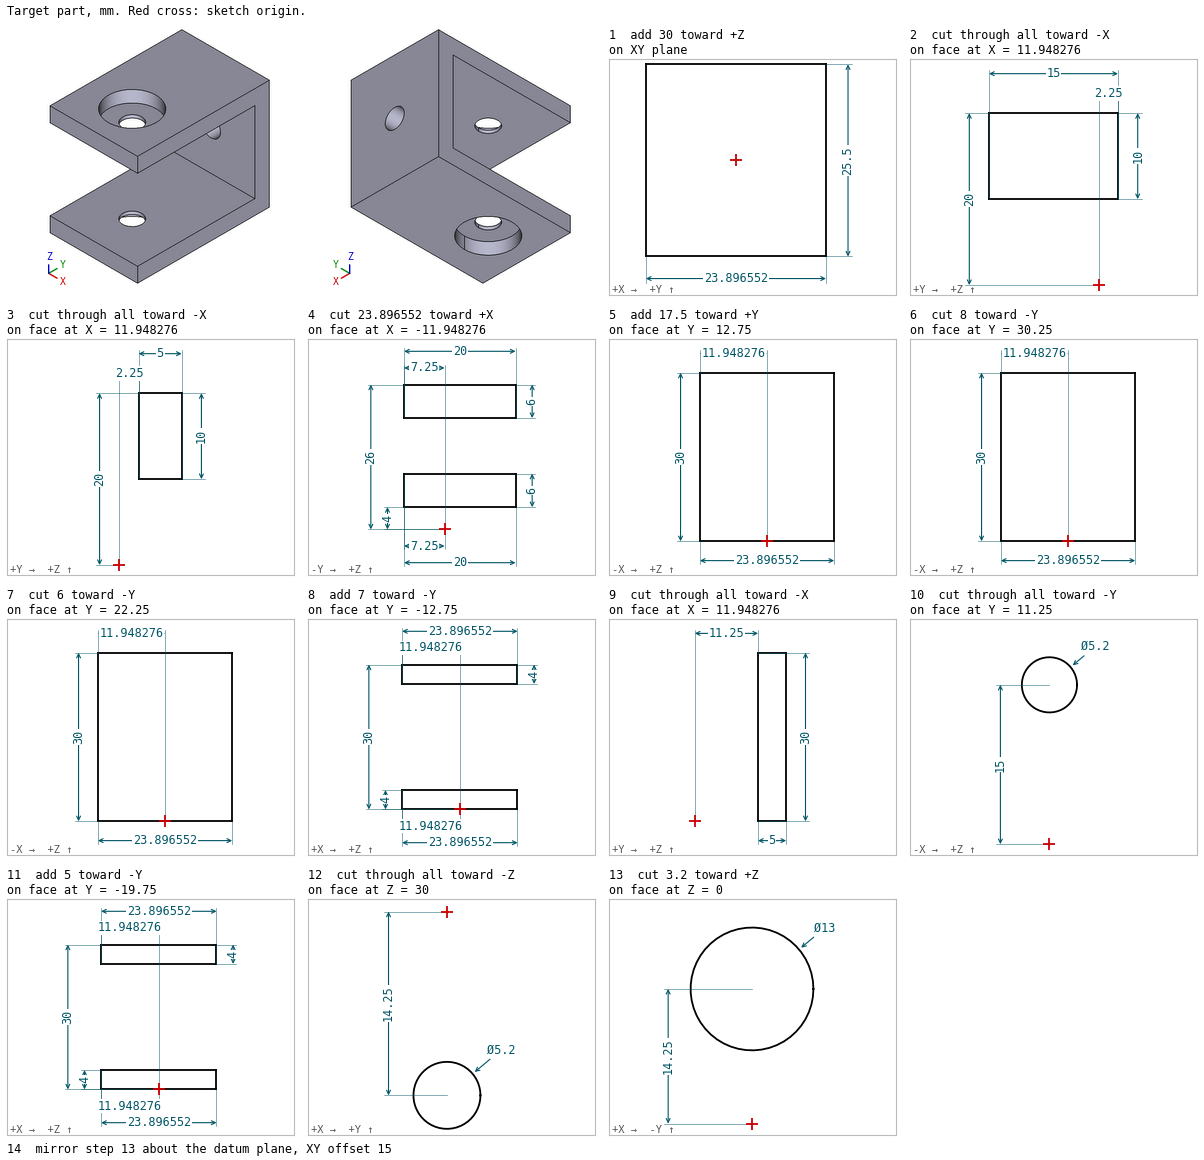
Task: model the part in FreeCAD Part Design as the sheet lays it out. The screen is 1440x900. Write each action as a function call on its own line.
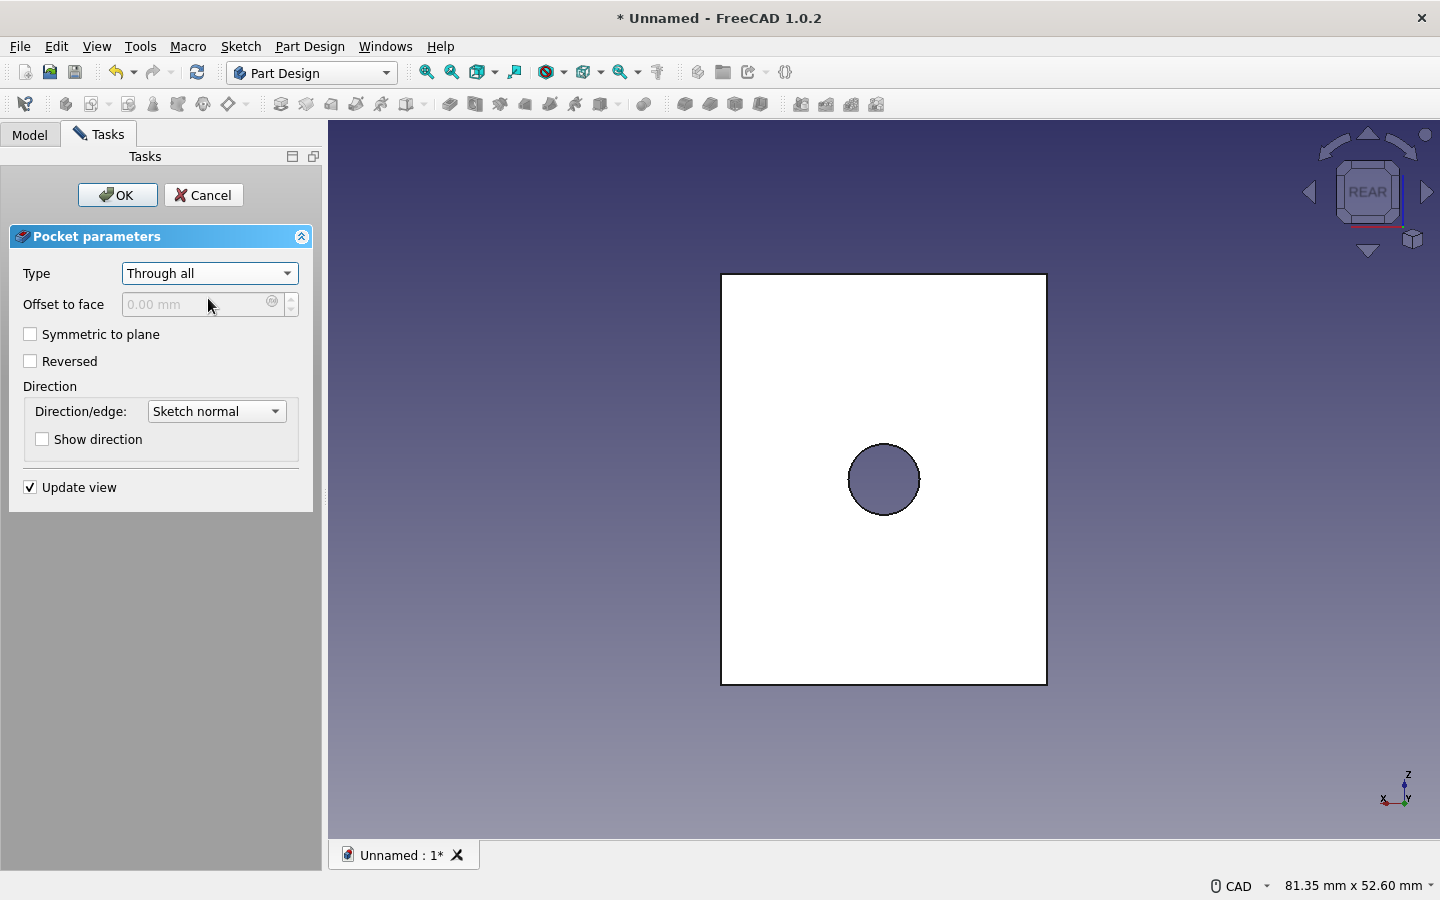
click(118, 195)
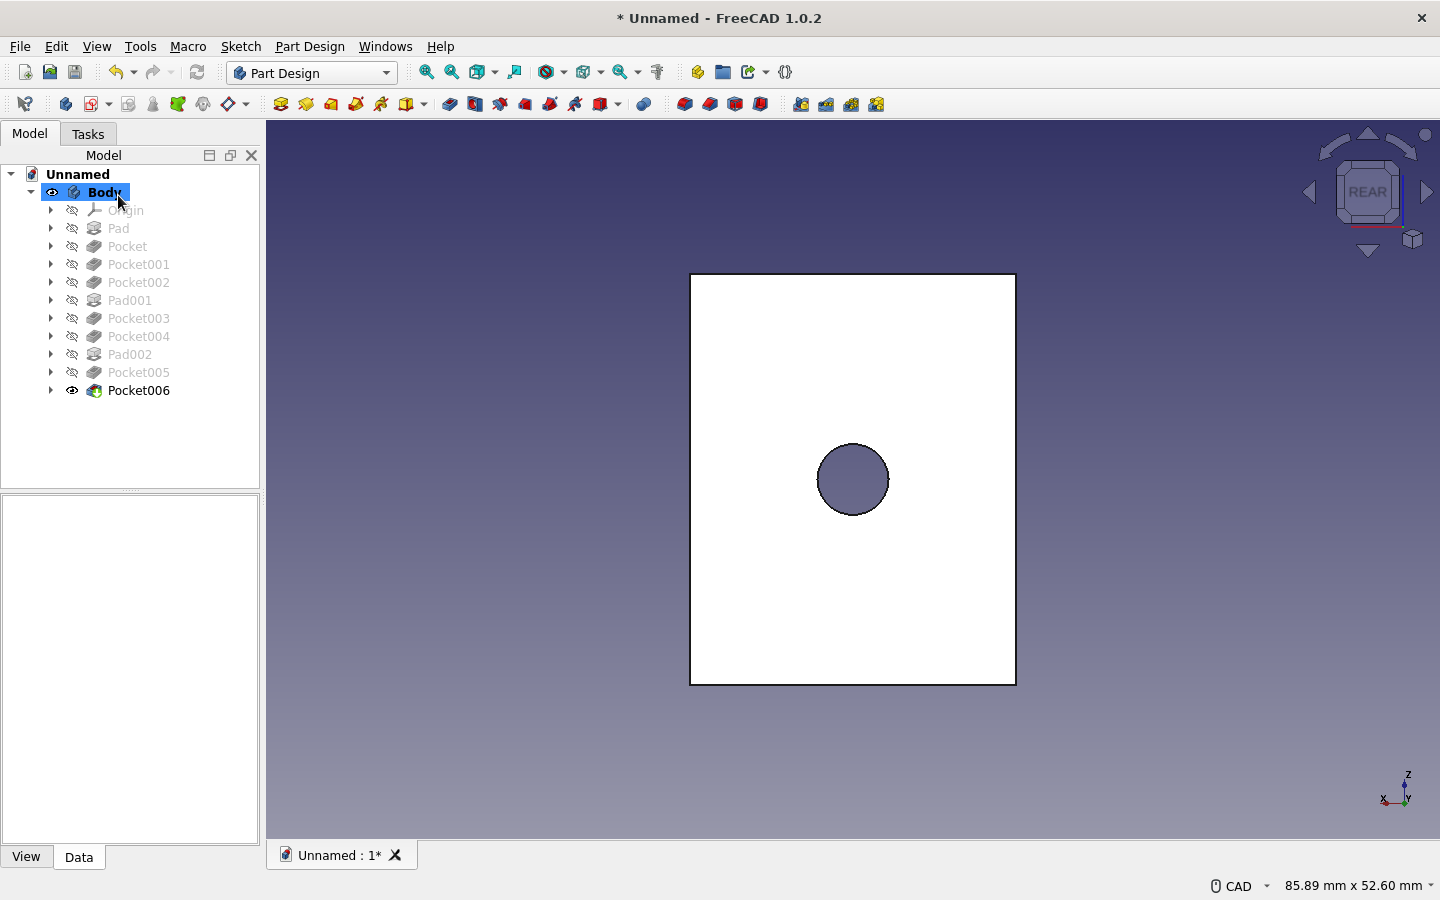
key(0)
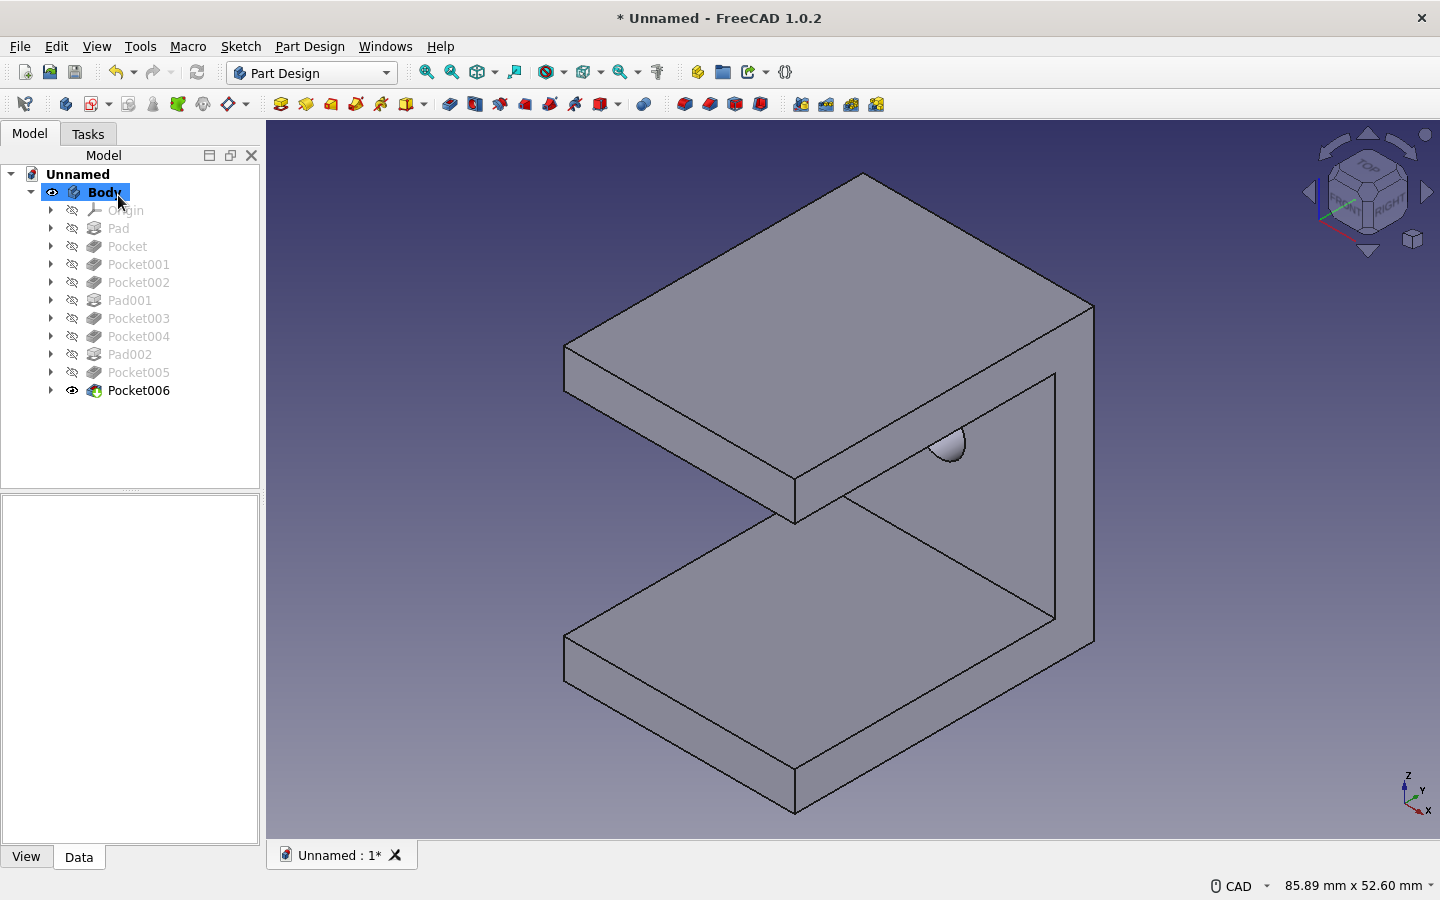
click(745, 472)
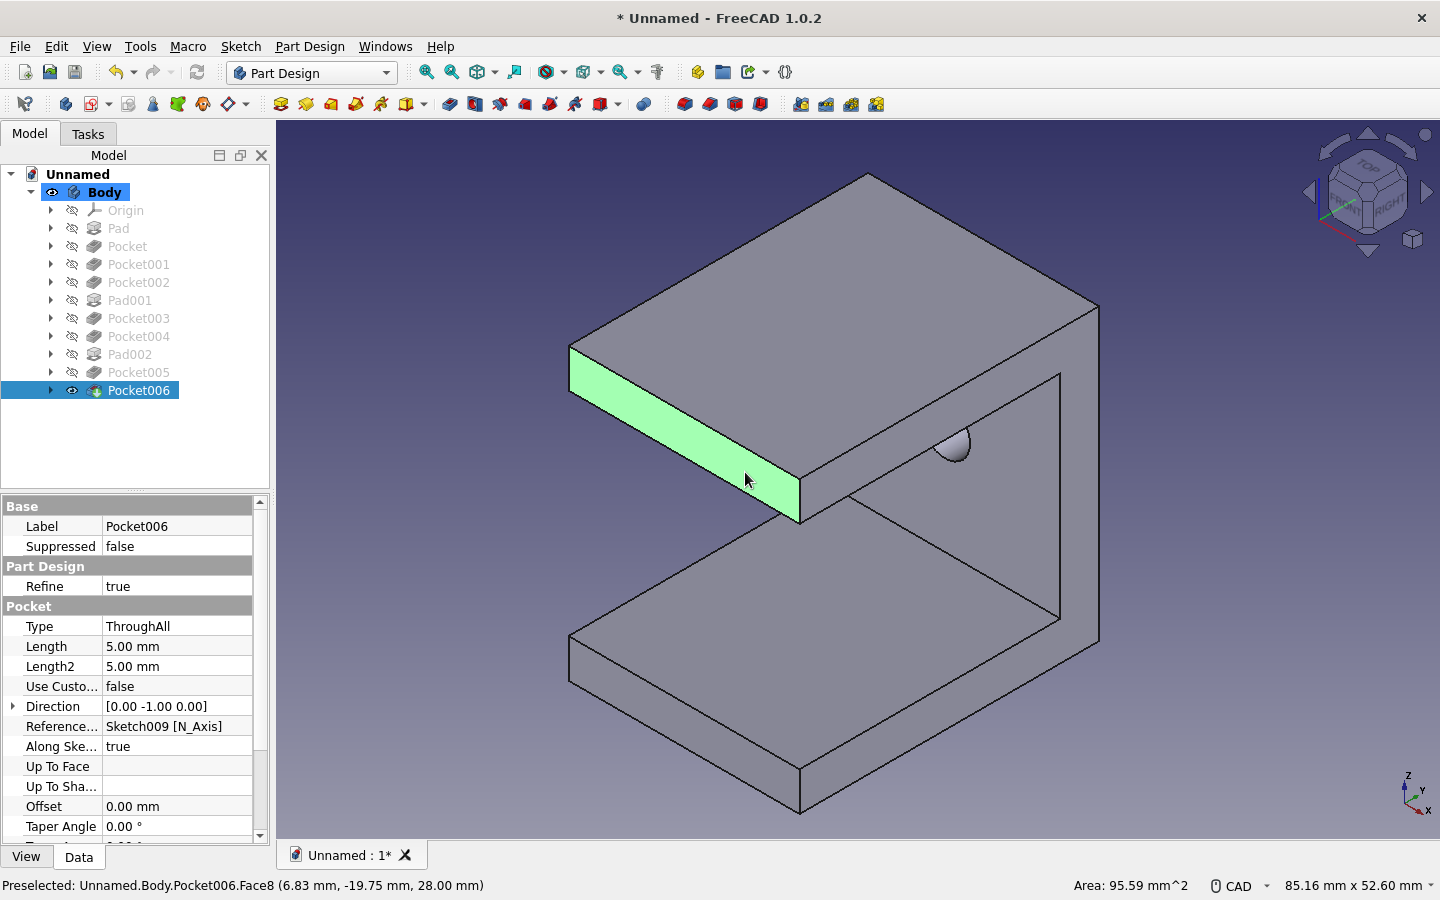
click(90, 104)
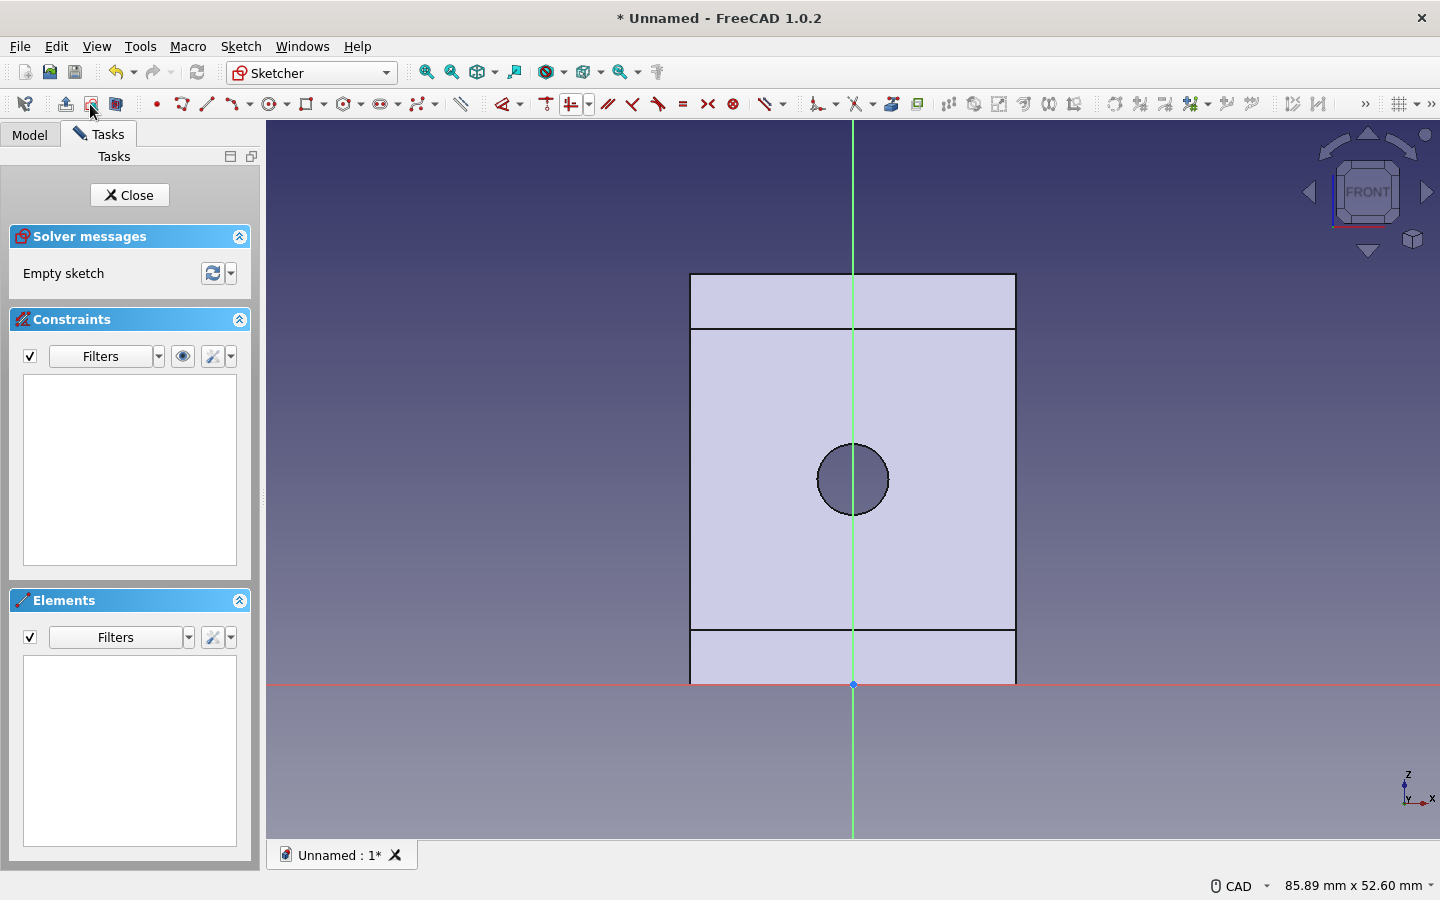
click(306, 104)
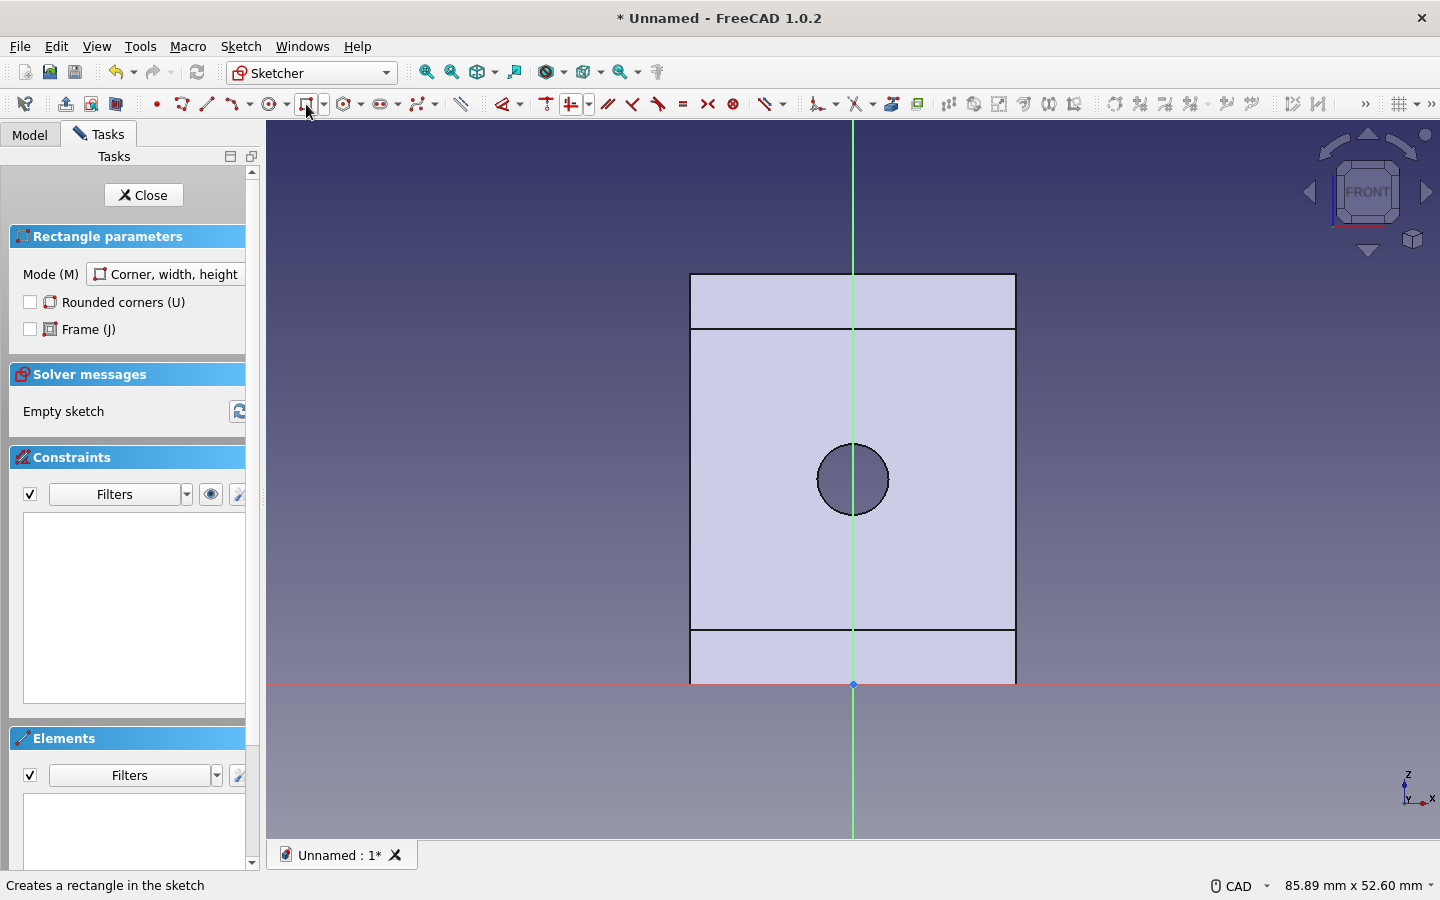
click(690, 630)
click(1016, 685)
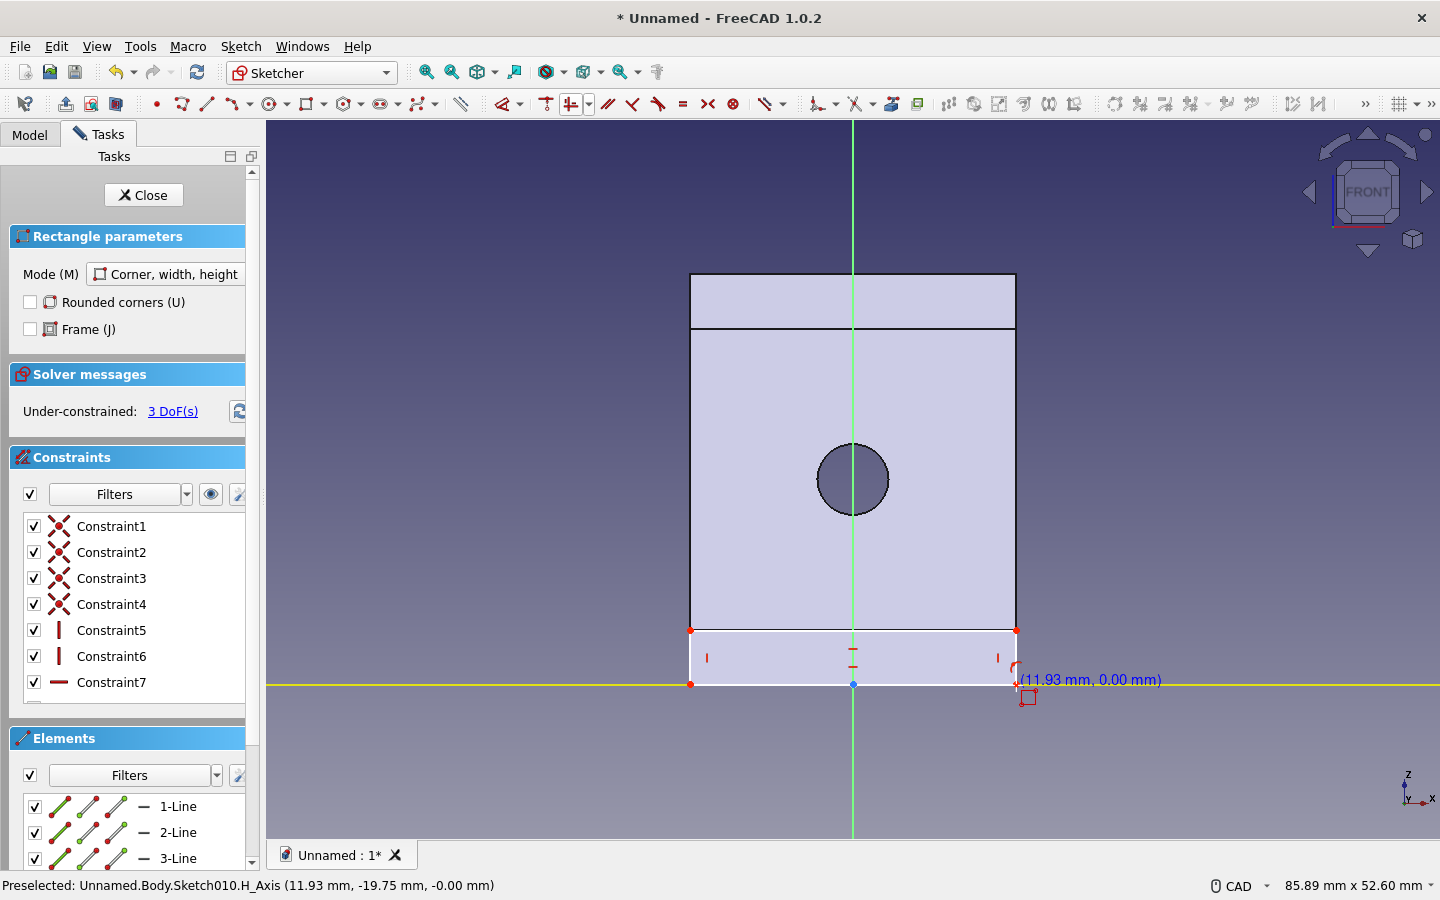
click(690, 274)
move(1016, 329)